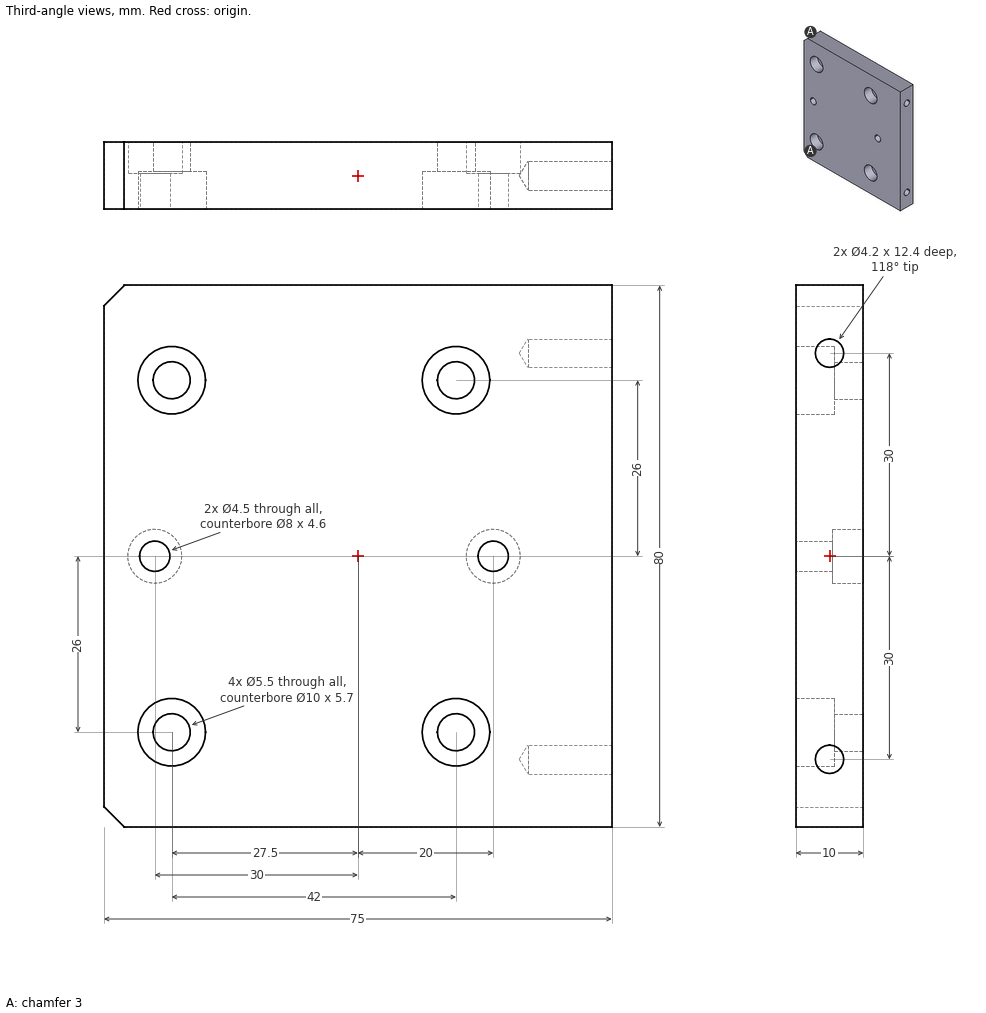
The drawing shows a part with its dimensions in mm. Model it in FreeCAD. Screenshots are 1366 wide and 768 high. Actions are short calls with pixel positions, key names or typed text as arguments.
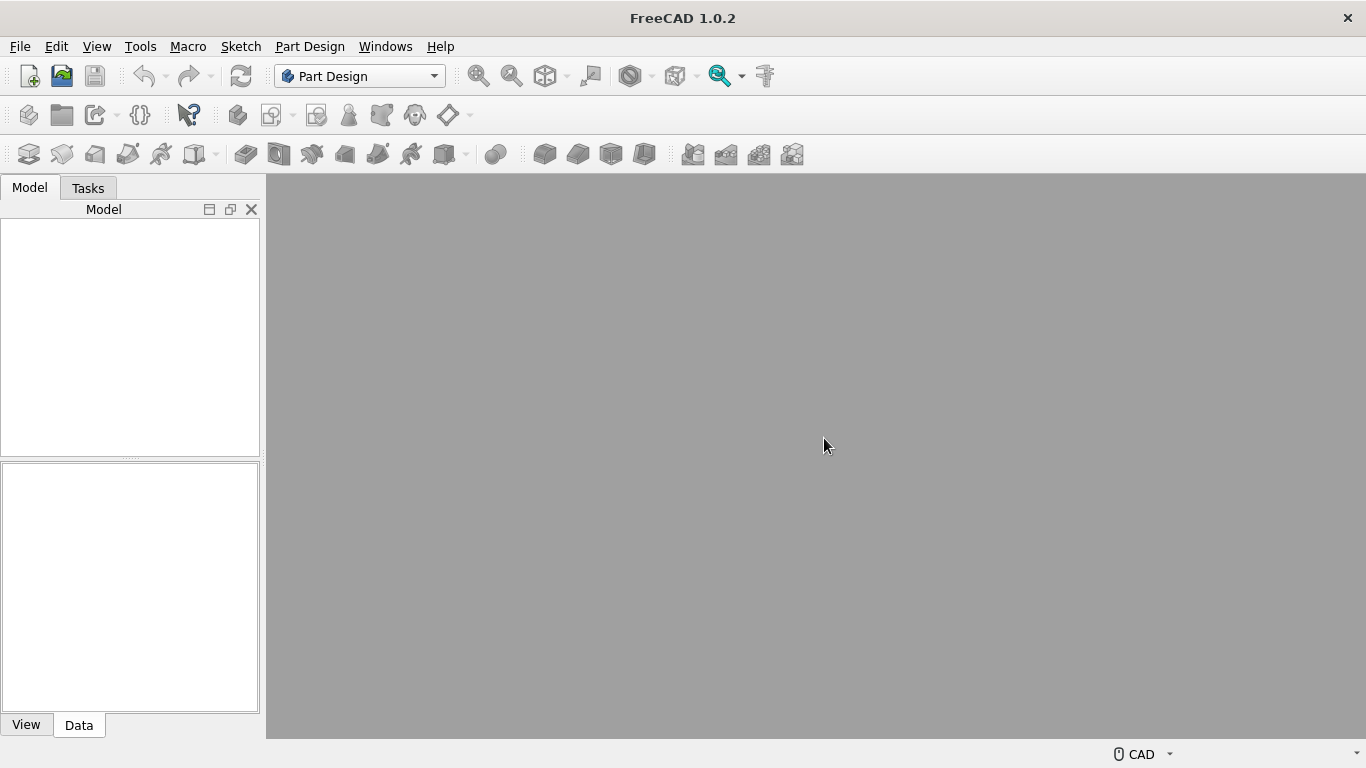
click(29, 76)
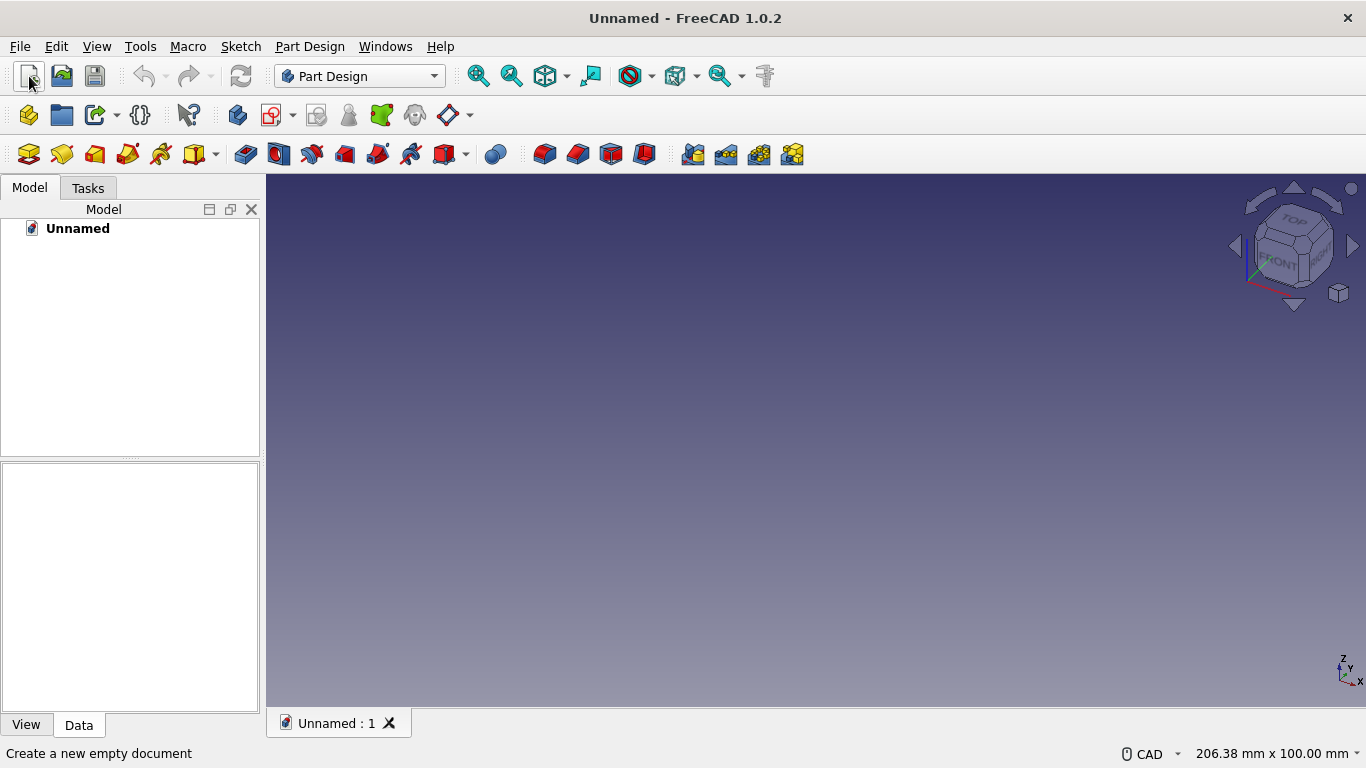
click(270, 116)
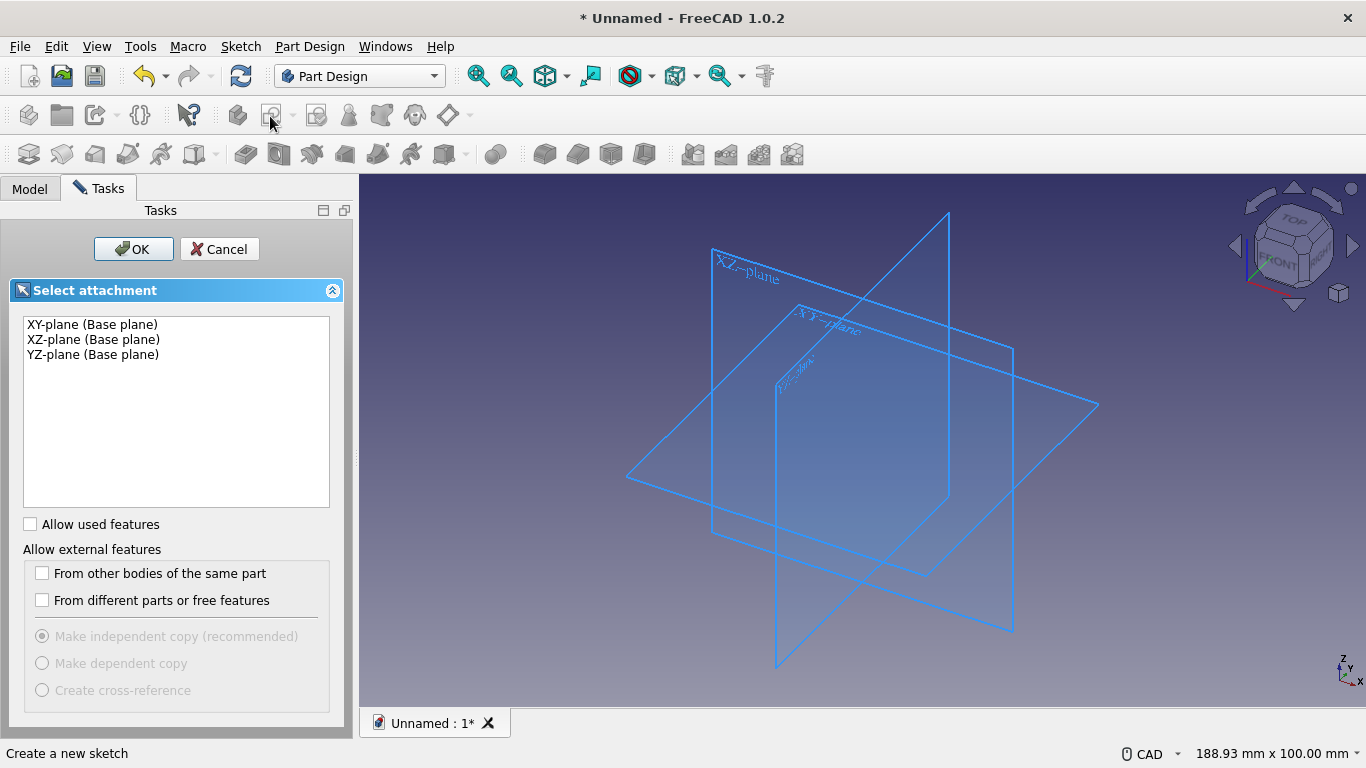
click(84, 340)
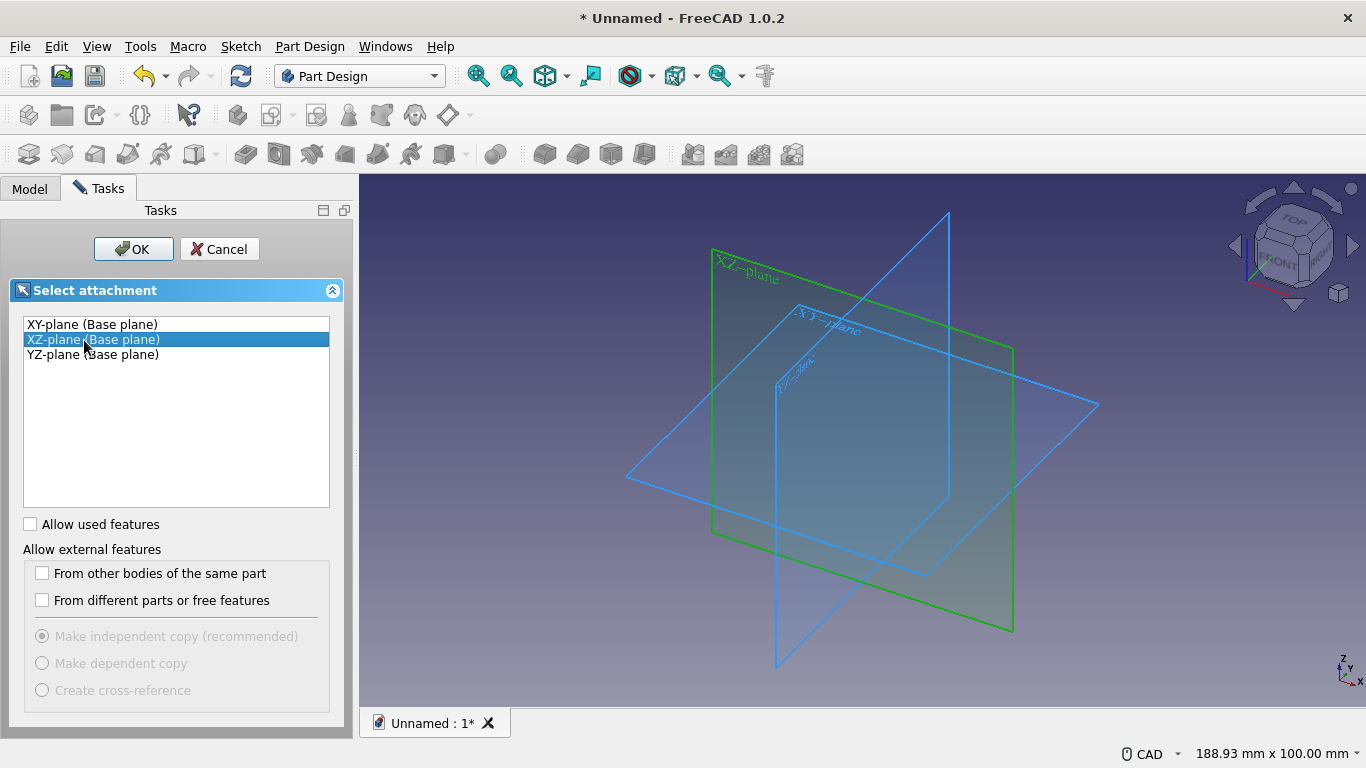
click(134, 249)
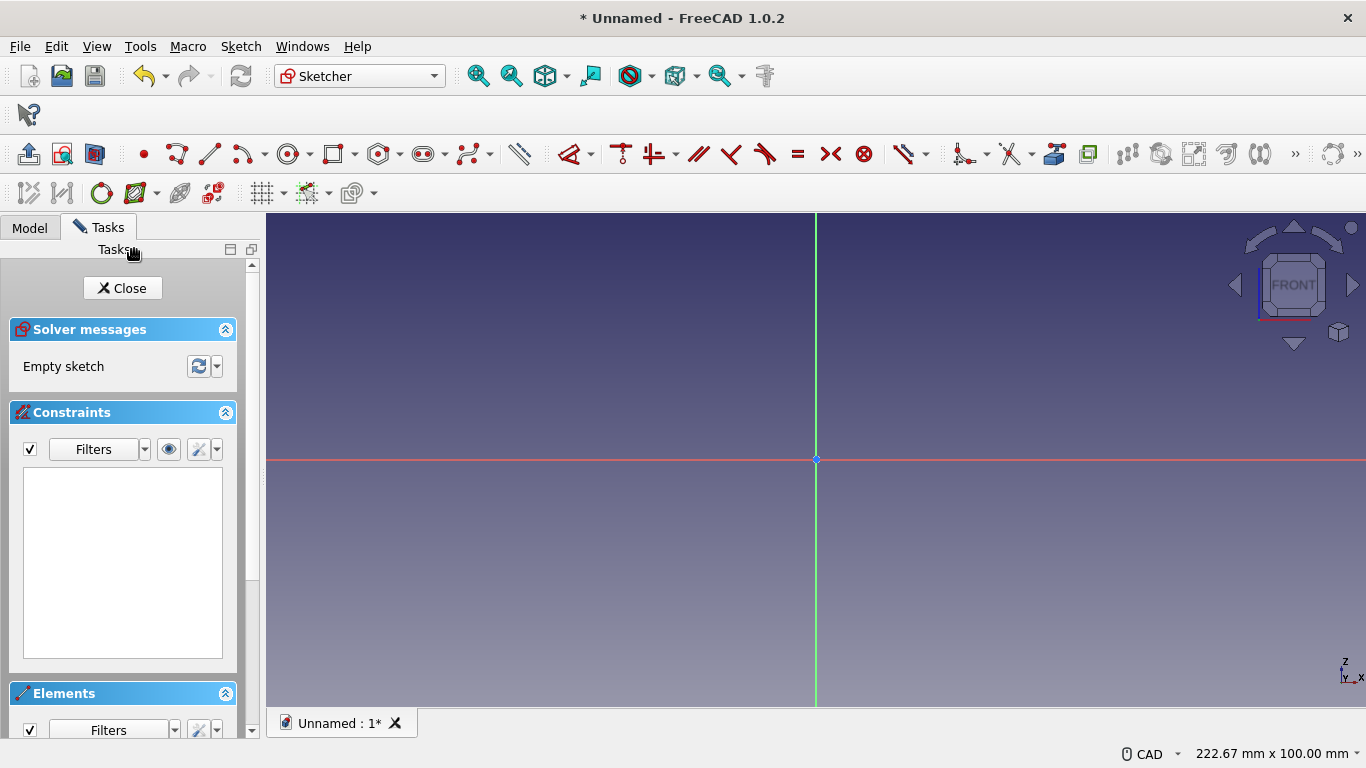
scroll(438, 460, down, 1)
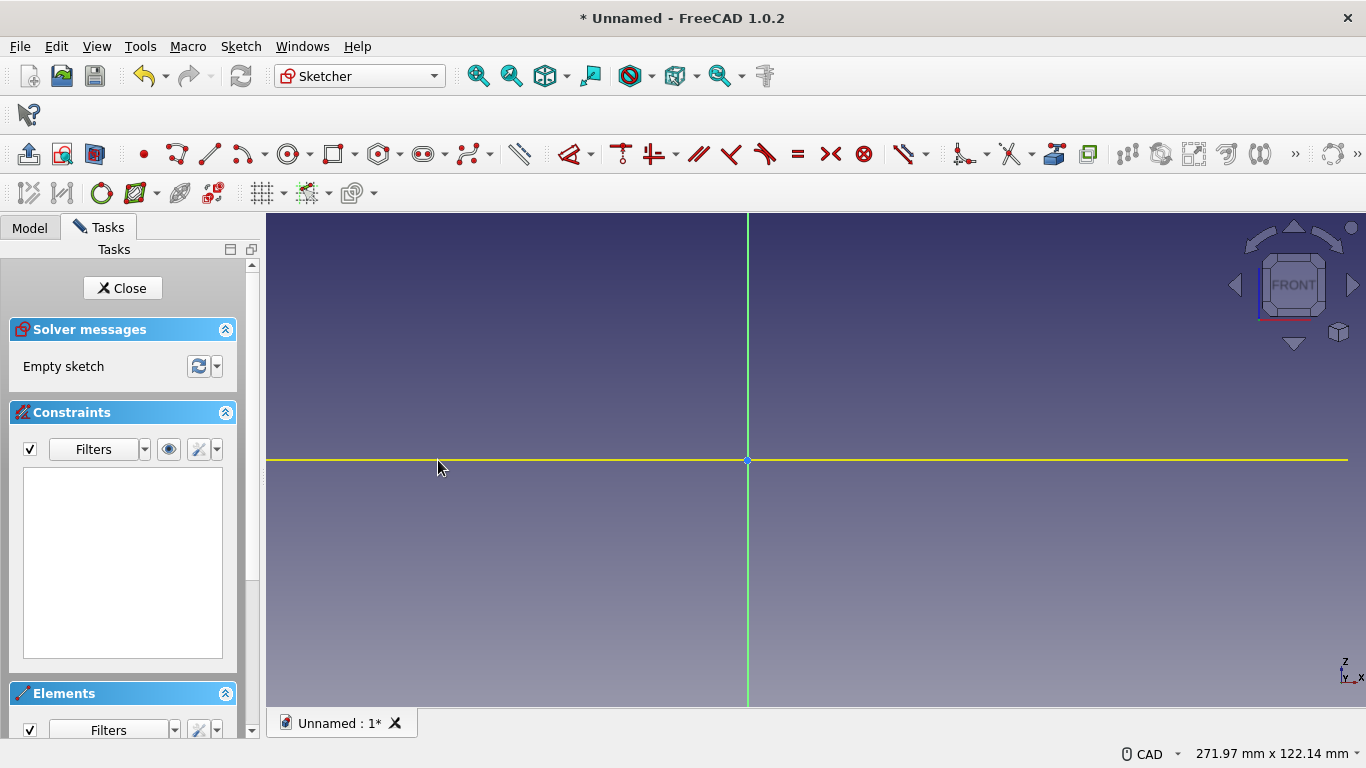
key(g)
key(v)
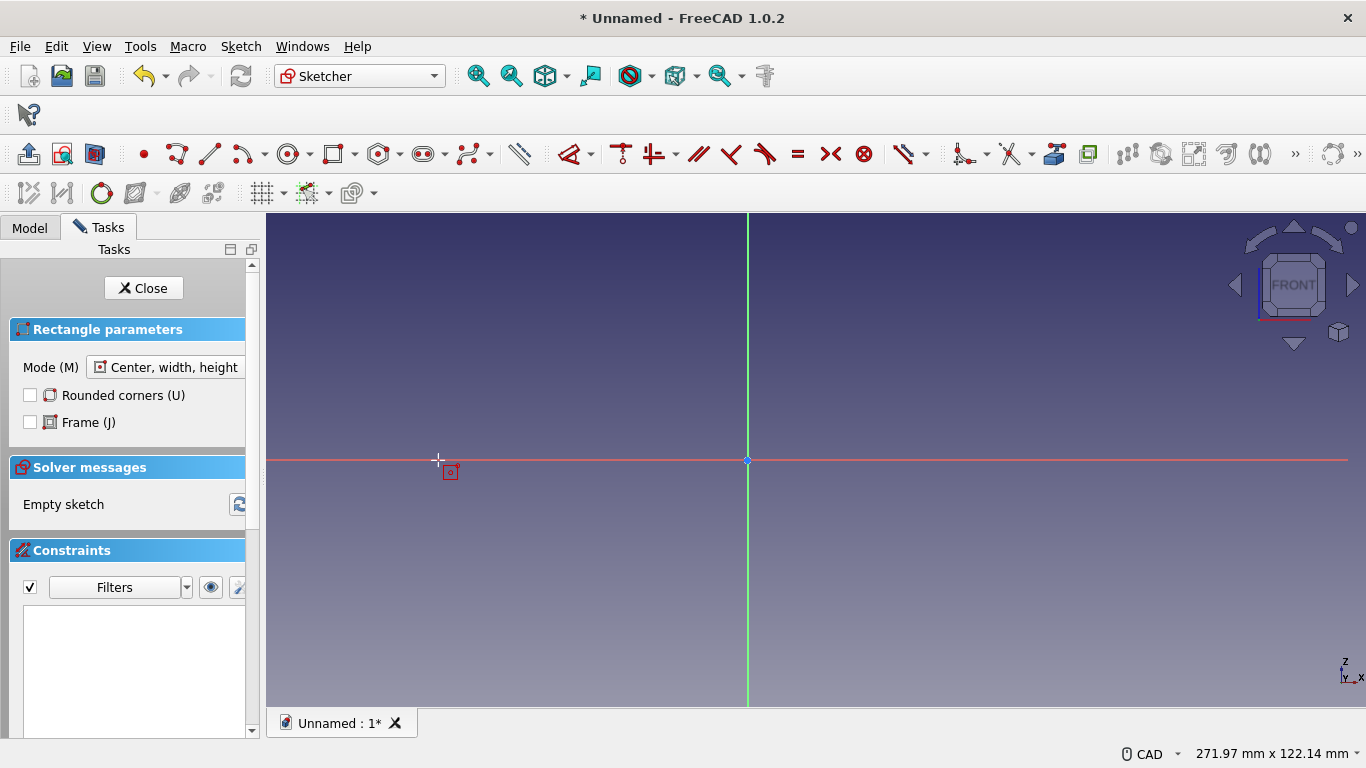
click(748, 460)
click(899, 298)
key(Escape)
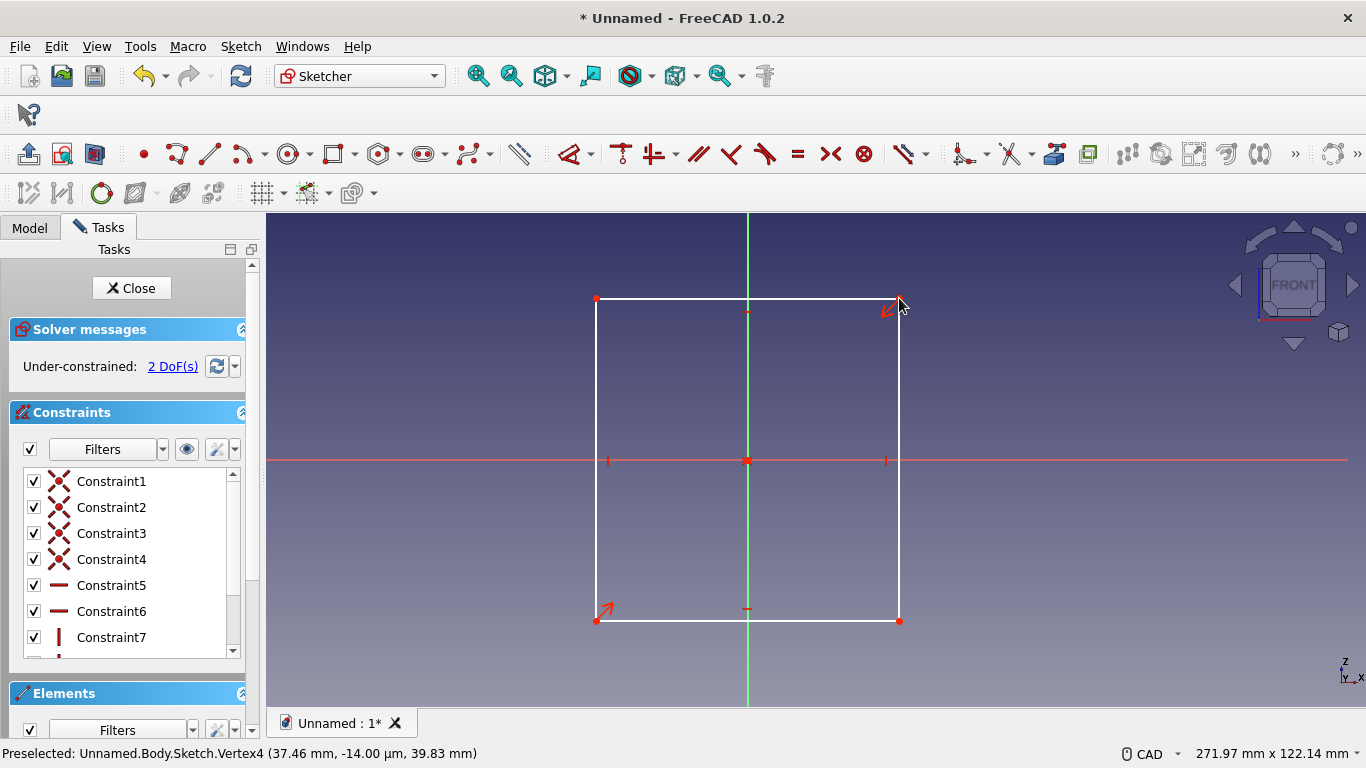
click(568, 154)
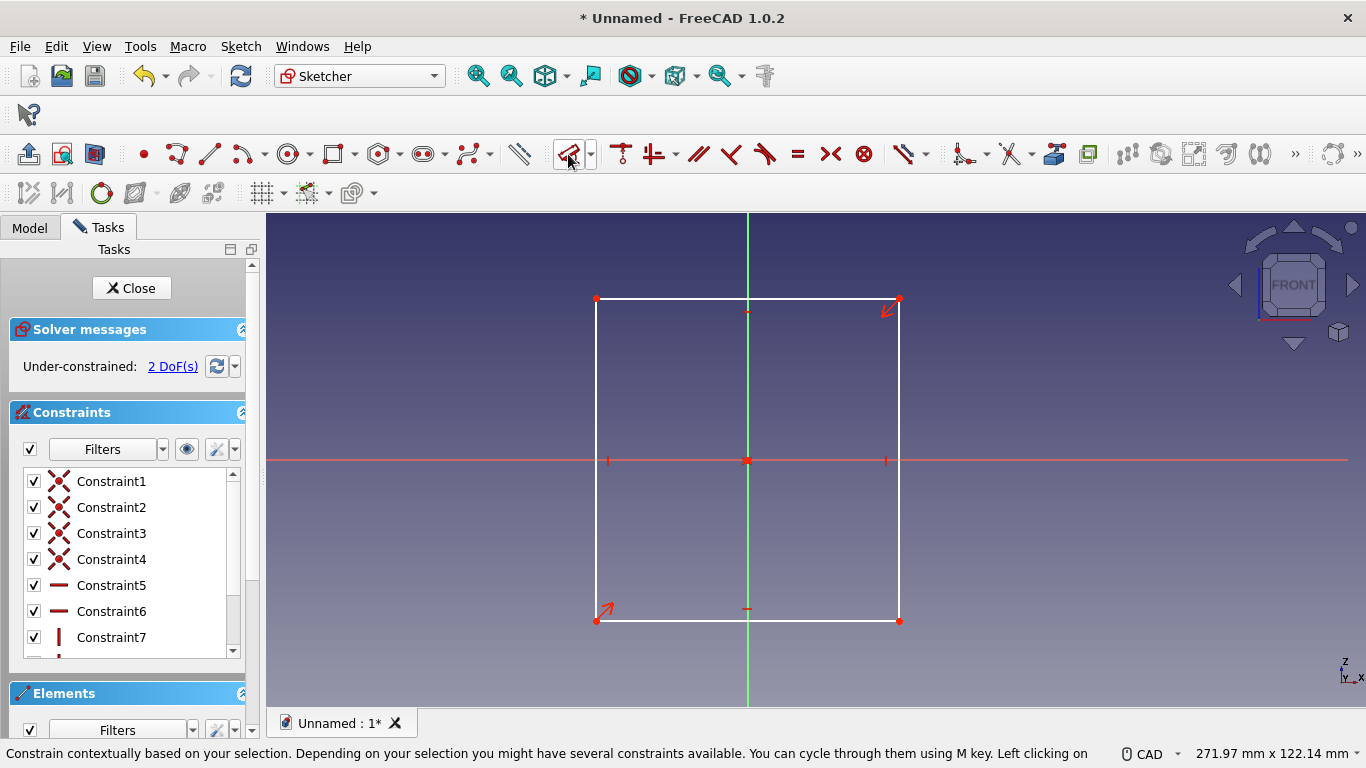
click(687, 621)
click(678, 655)